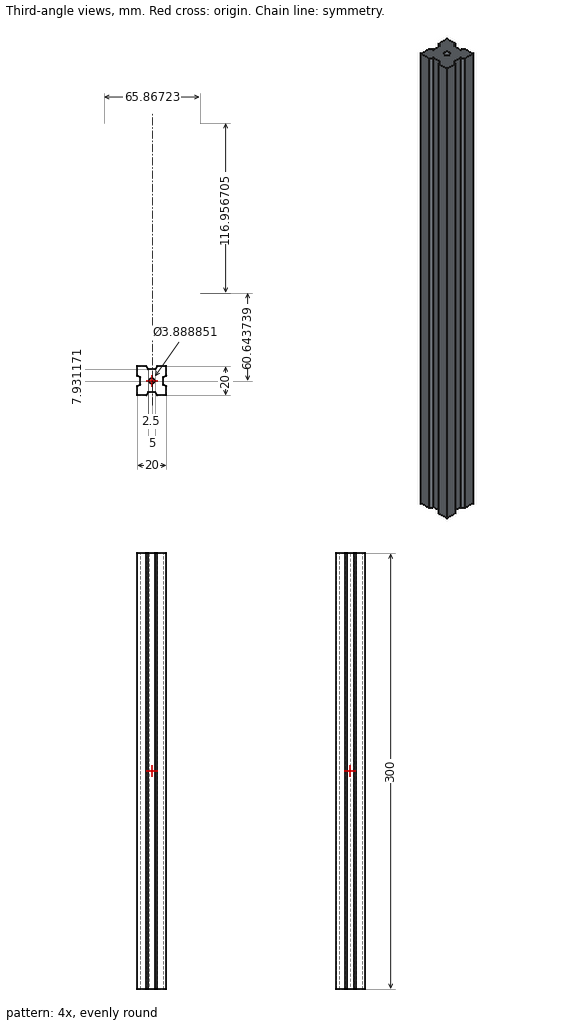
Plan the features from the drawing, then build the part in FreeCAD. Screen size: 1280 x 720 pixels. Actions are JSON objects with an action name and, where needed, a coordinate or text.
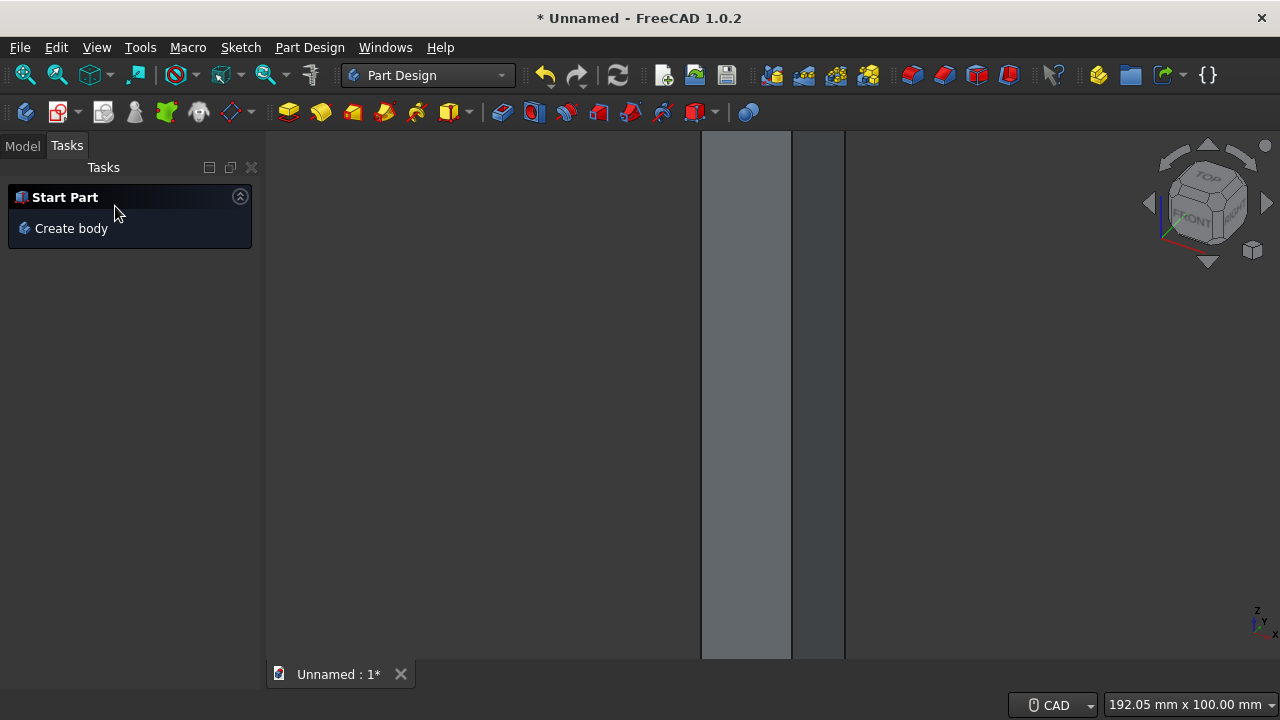
{"action": "left_click", "coordinate": [26, 76]}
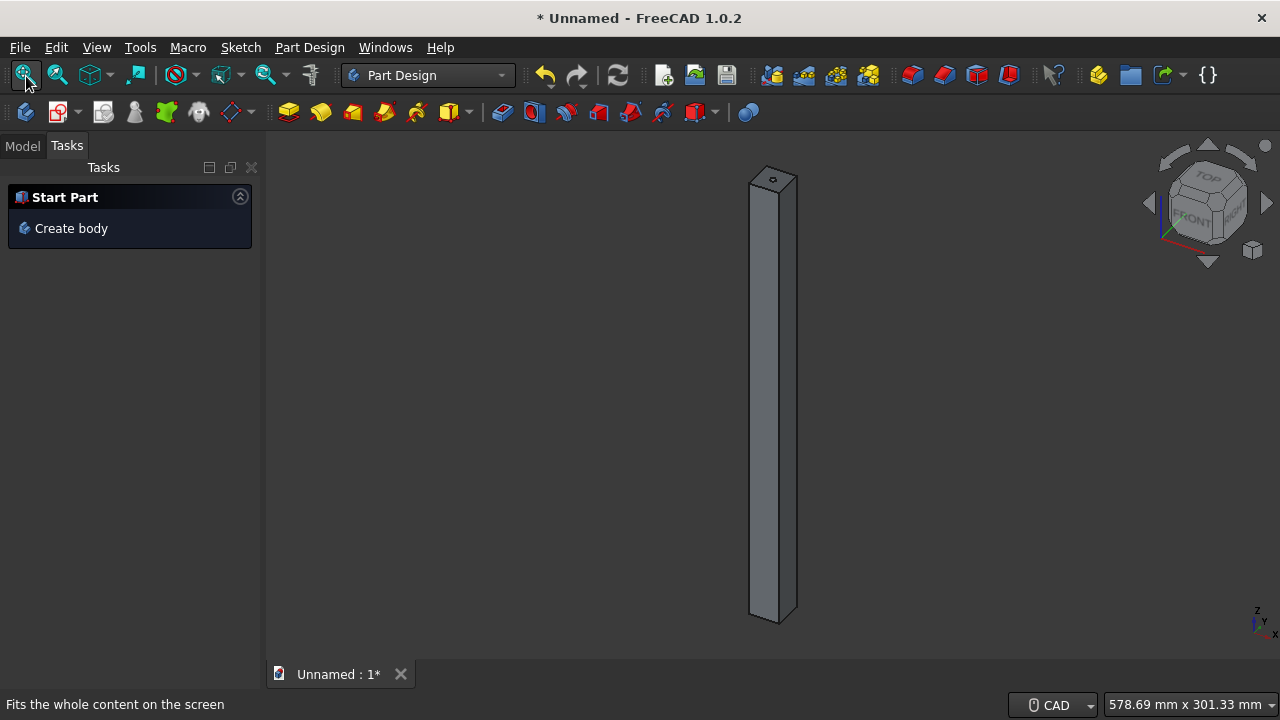
{"action": "key", "text": "0"}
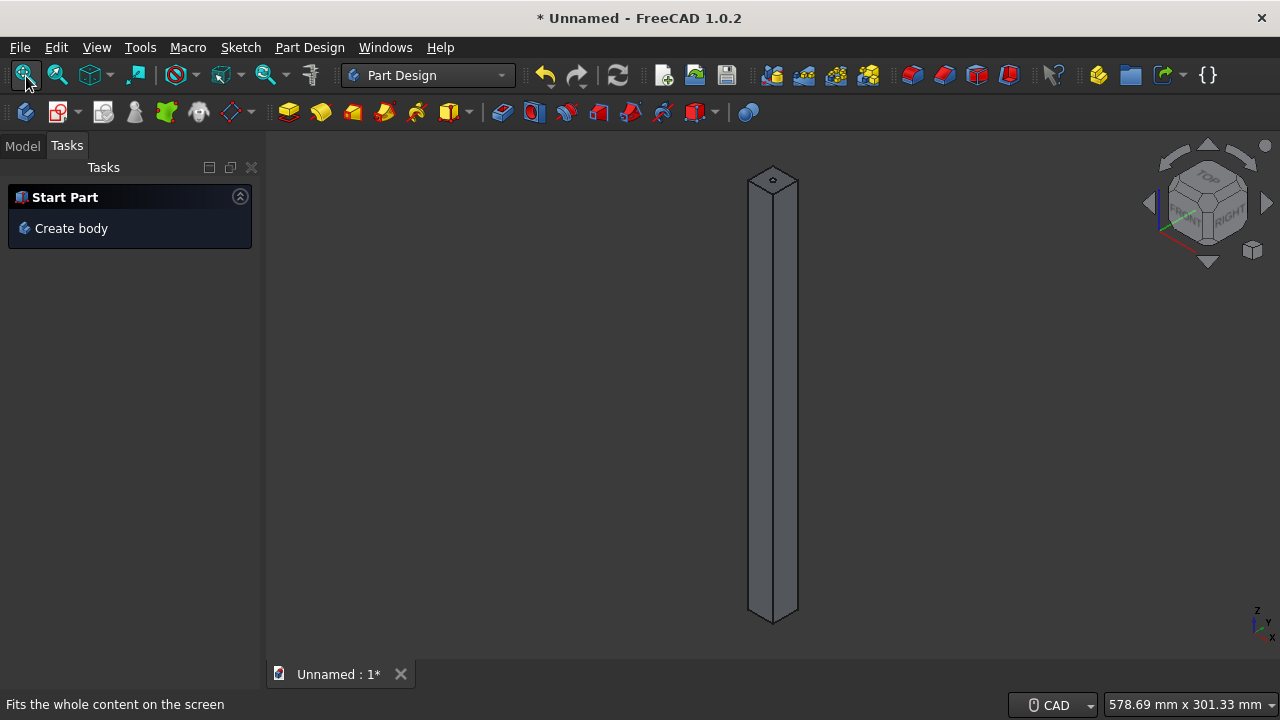
{"action": "key", "text": "2"}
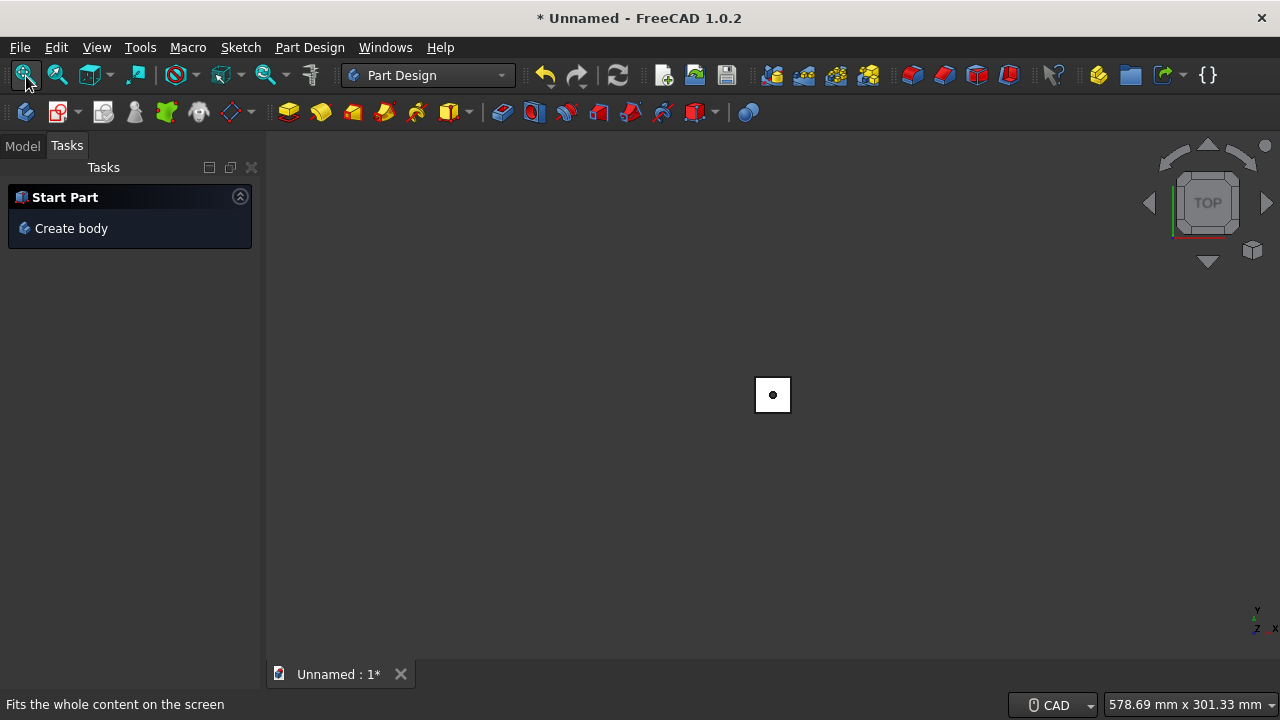
{"action": "left_click", "coordinate": [26, 76]}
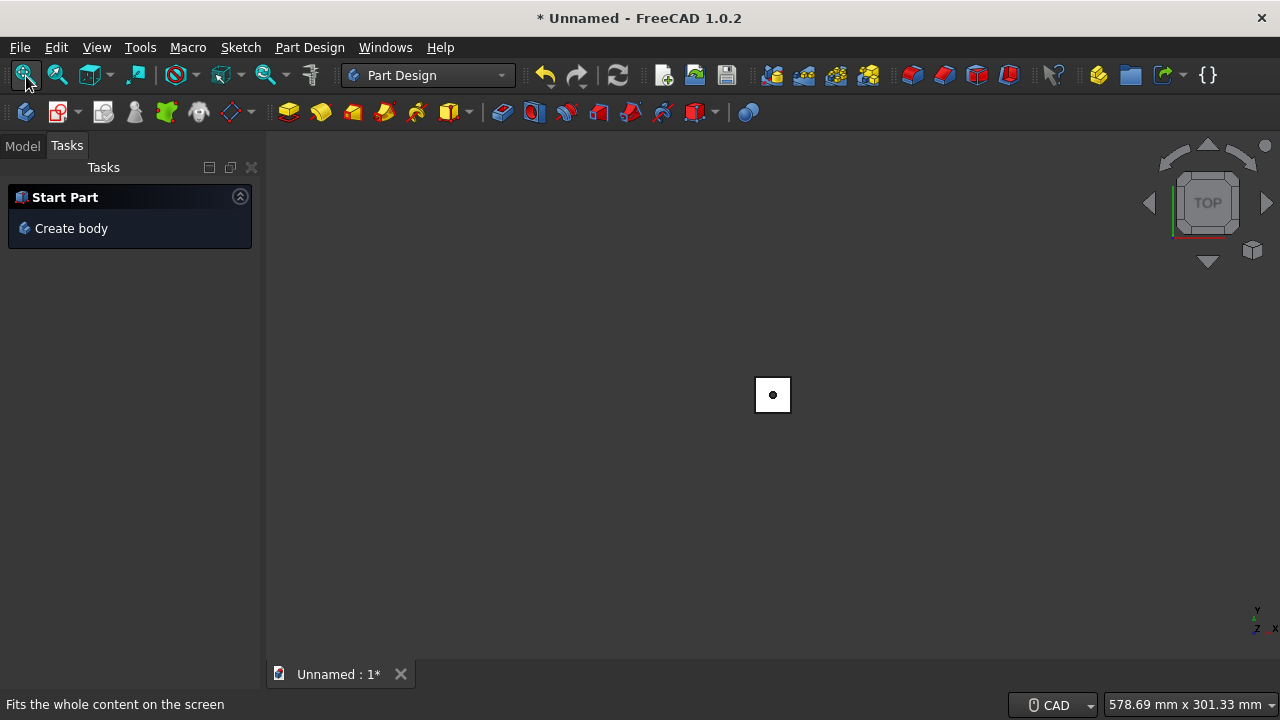
{"action": "key", "text": "1"}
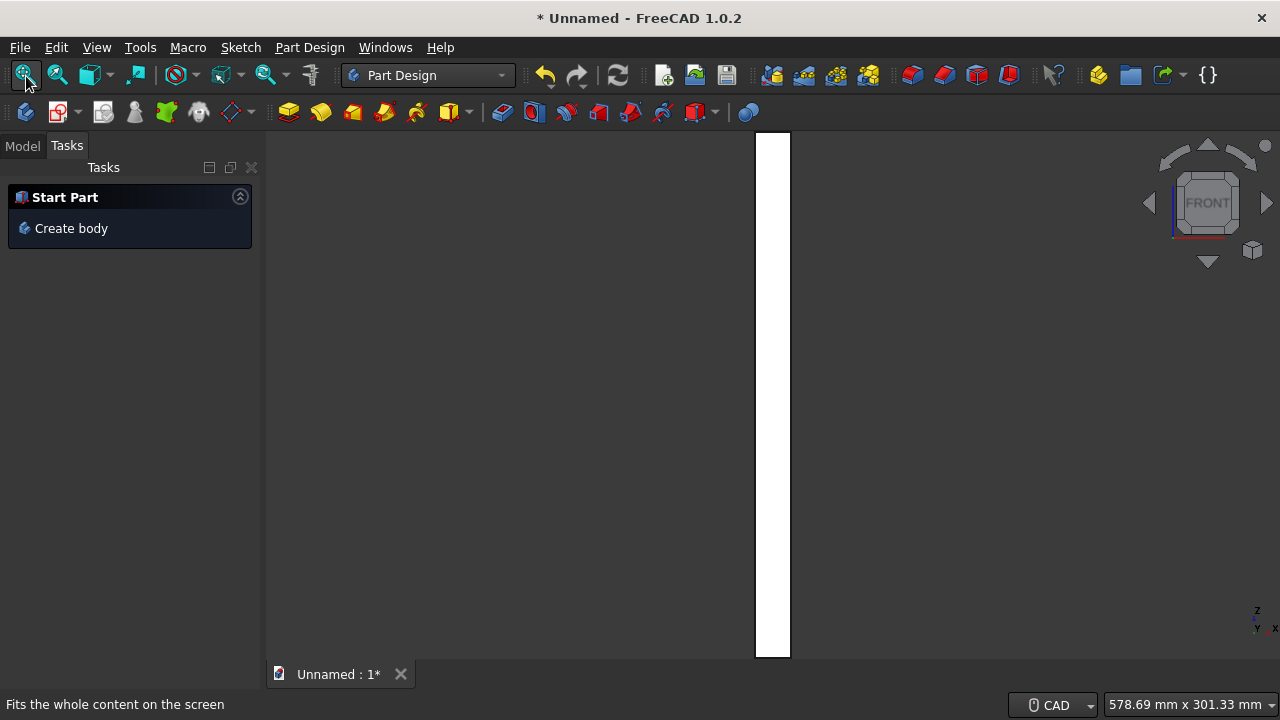
{"action": "left_click", "coordinate": [23, 145]}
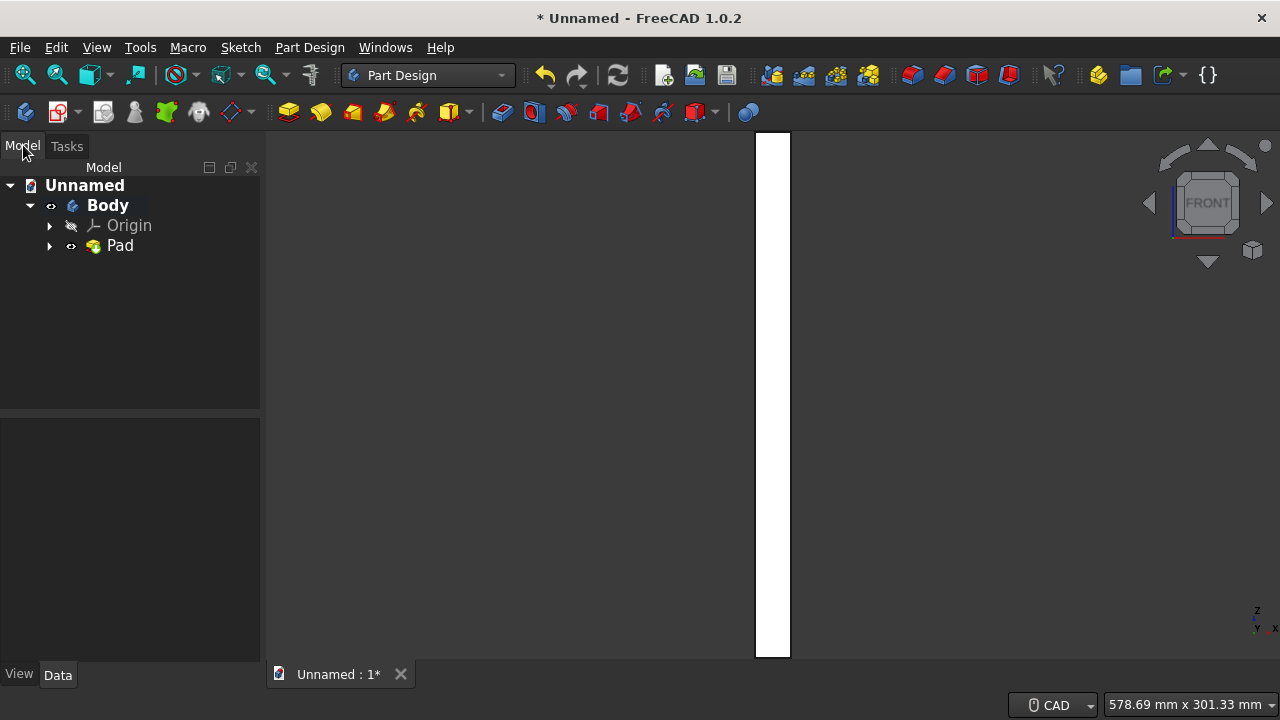
{"action": "left_click", "coordinate": [50, 226]}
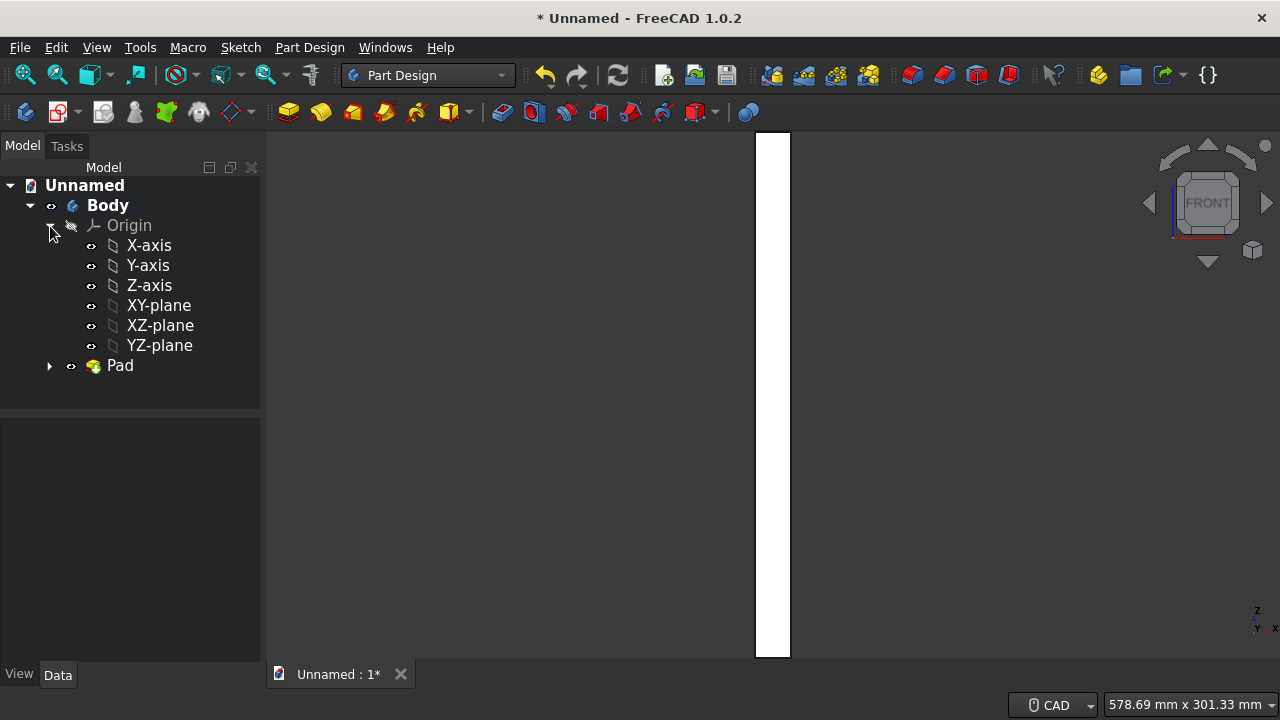
{"action": "left_click", "coordinate": [136, 306]}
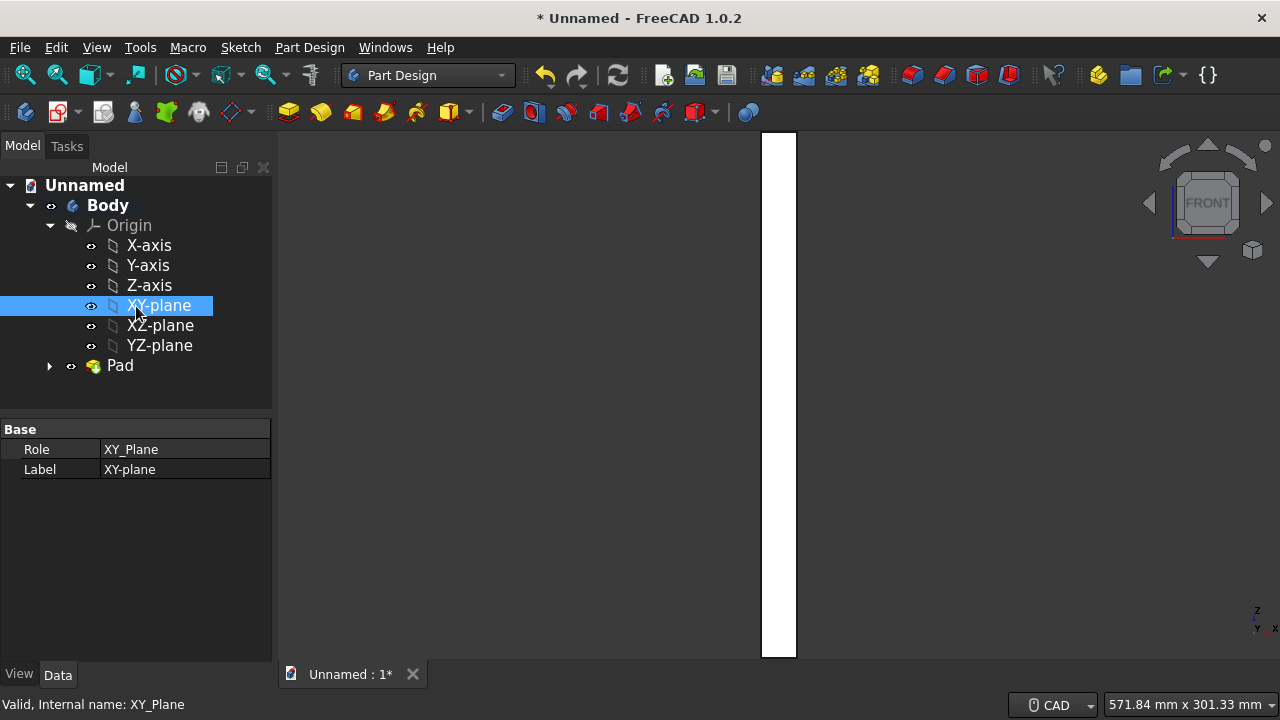
{"action": "left_click", "coordinate": [232, 112]}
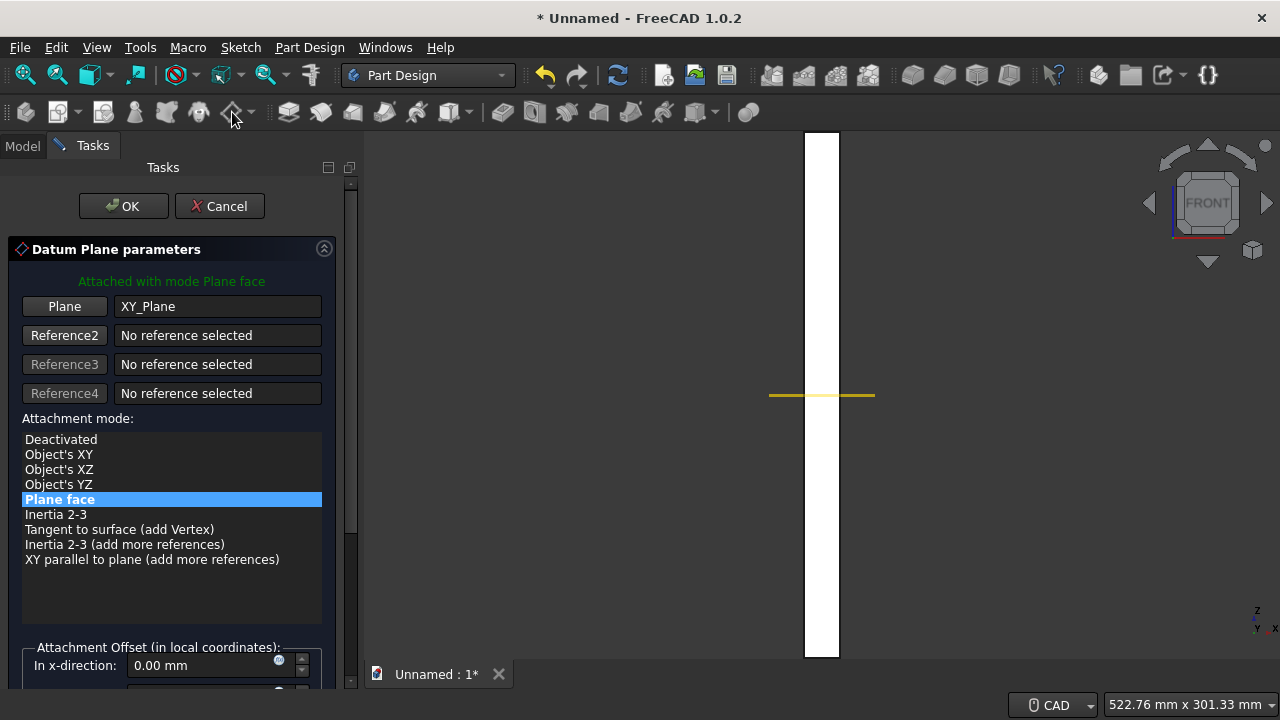
{"action": "scroll", "coordinate": [351, 432], "scroll_direction": "down", "scroll_amount": 2}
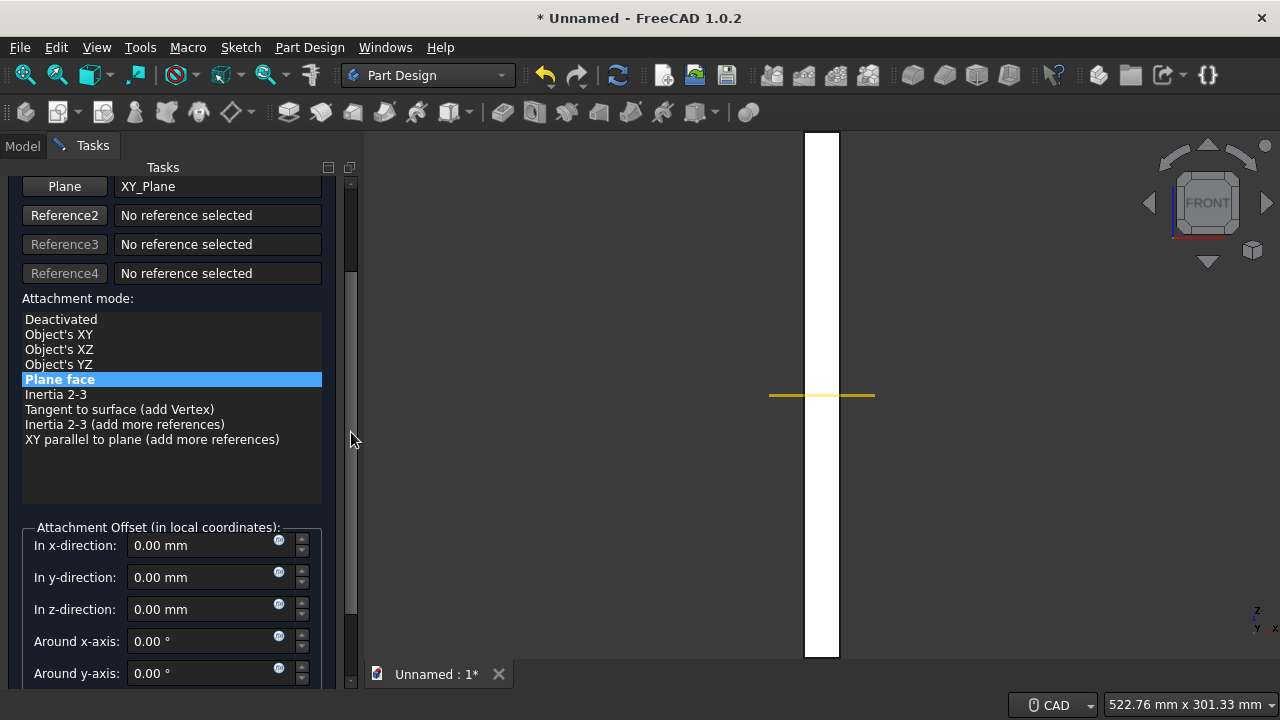
{"action": "triple_click", "coordinate": [210, 609]}